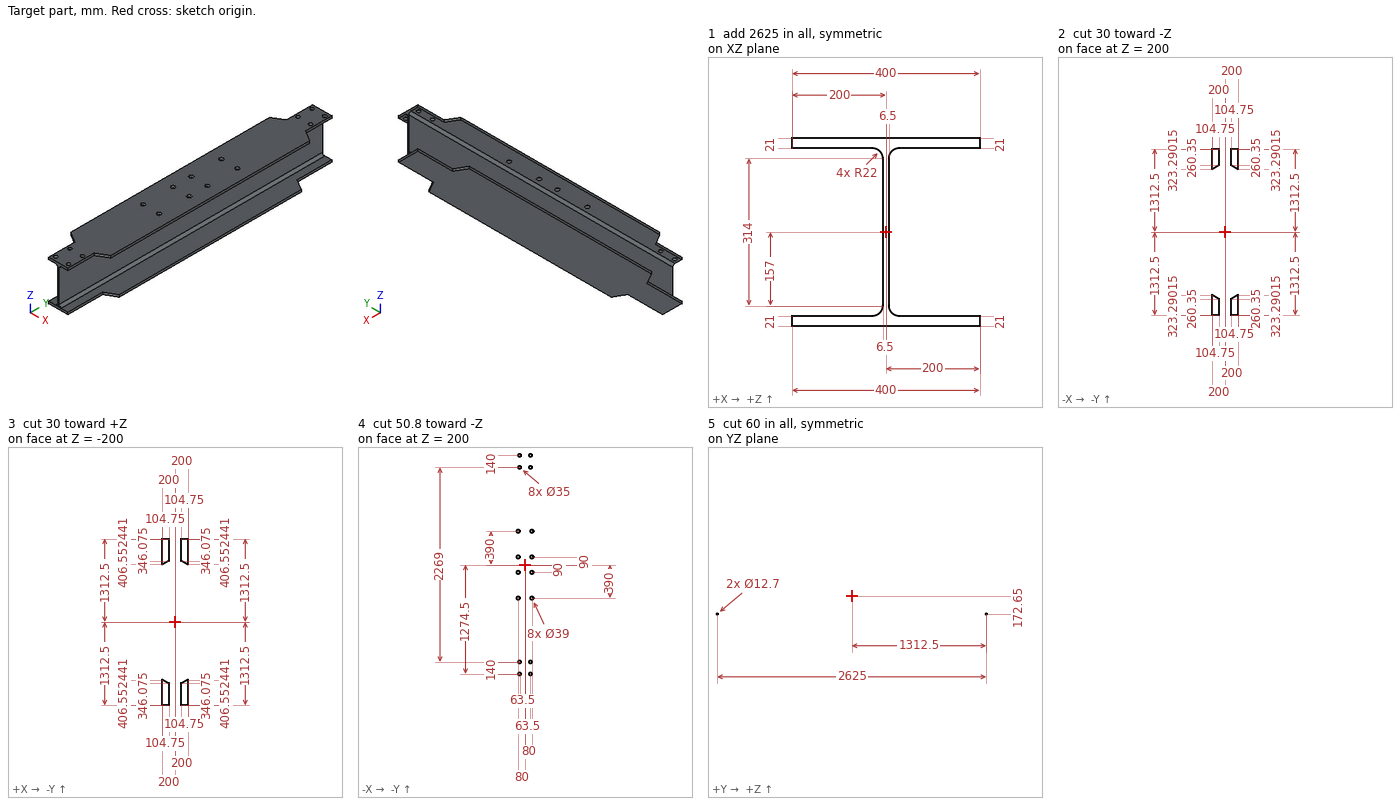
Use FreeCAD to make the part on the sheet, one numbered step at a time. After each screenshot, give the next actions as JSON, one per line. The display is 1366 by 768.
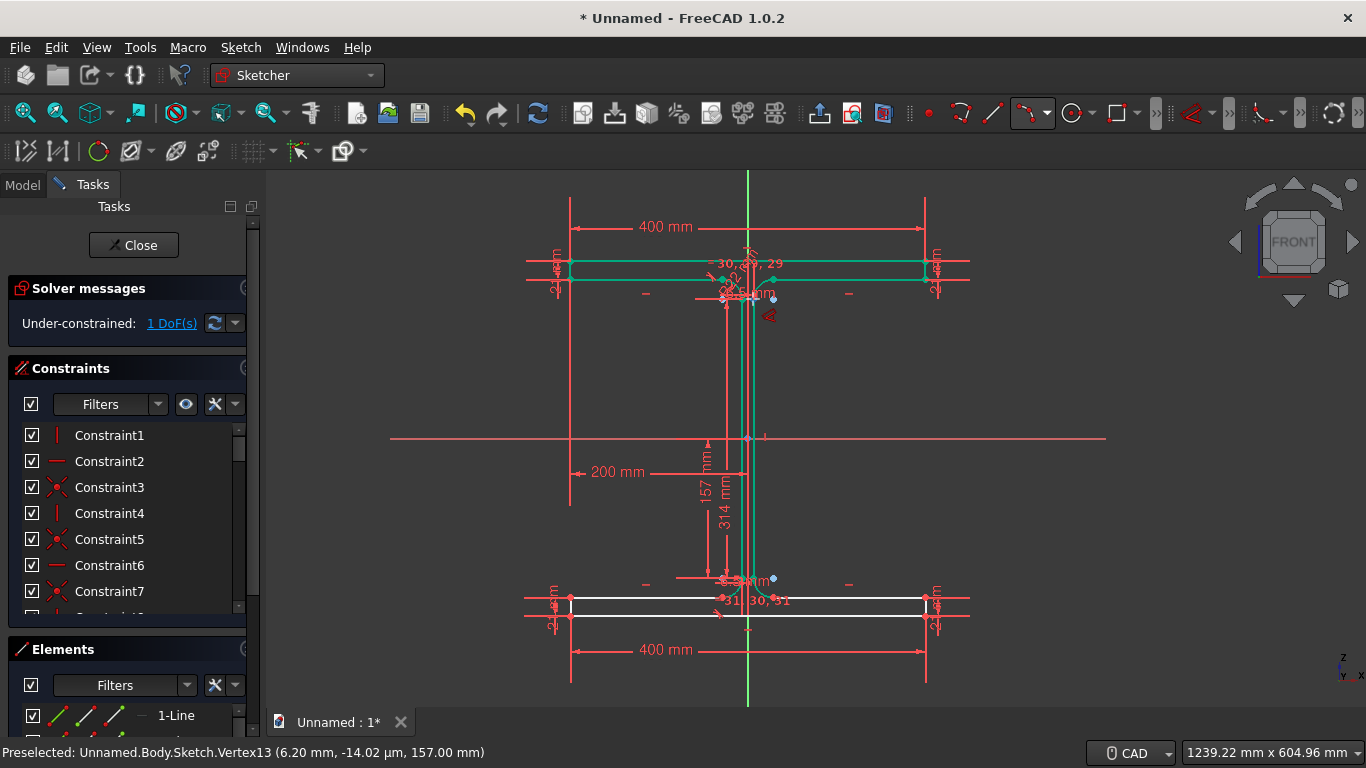
{"action": "left_click", "coordinate": [926, 598]}
{"action": "left_click", "coordinate": [837, 632]}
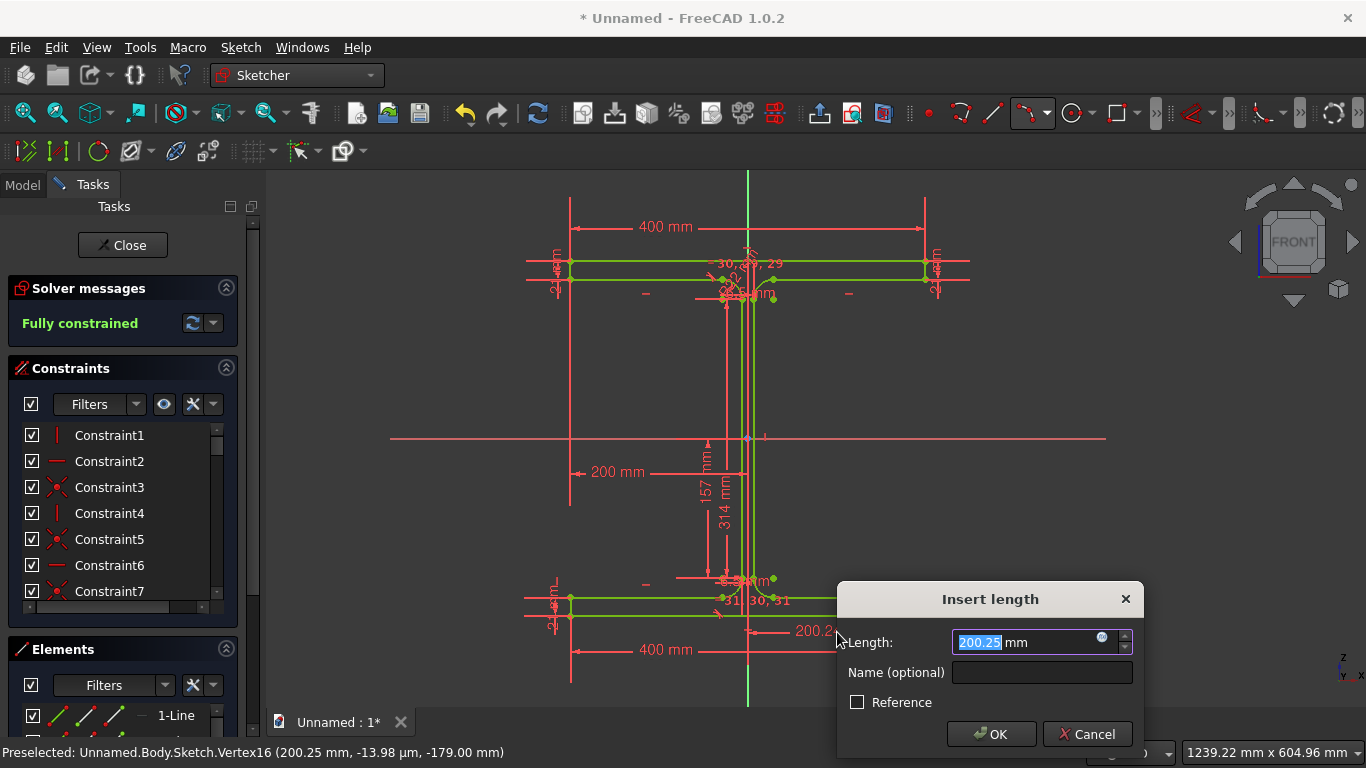
{"action": "type", "text": "200"}
{"action": "key", "text": "Return"}
{"action": "key", "text": "Escape"}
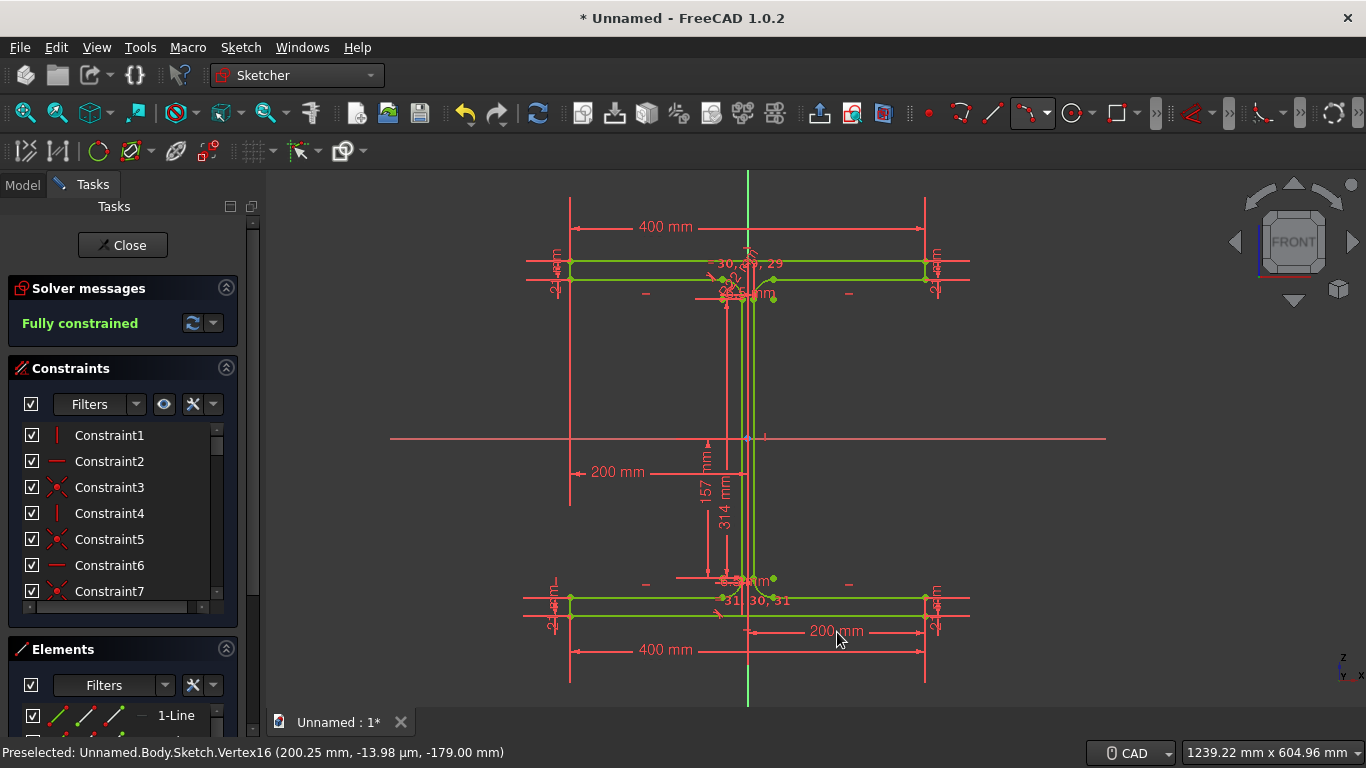
{"action": "left_click", "coordinate": [123, 245]}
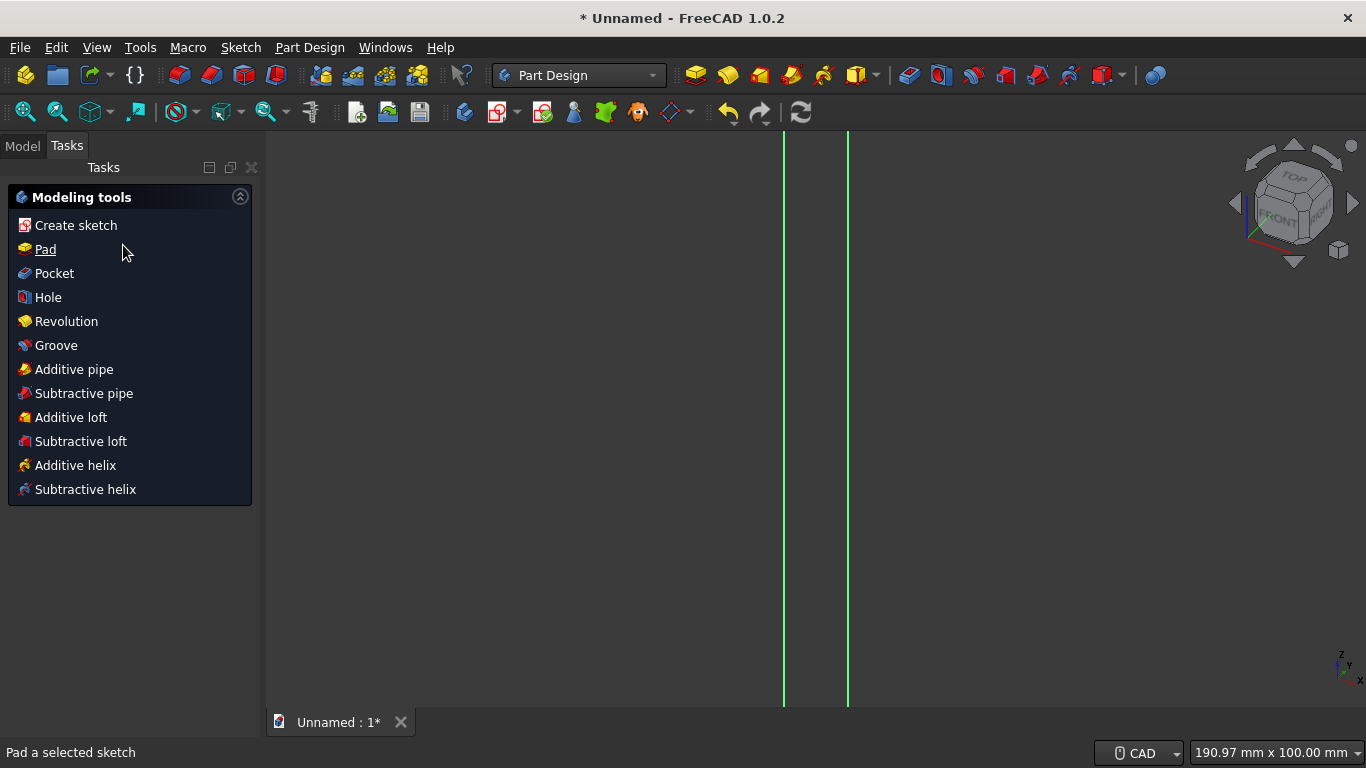
{"action": "left_click", "coordinate": [696, 76]}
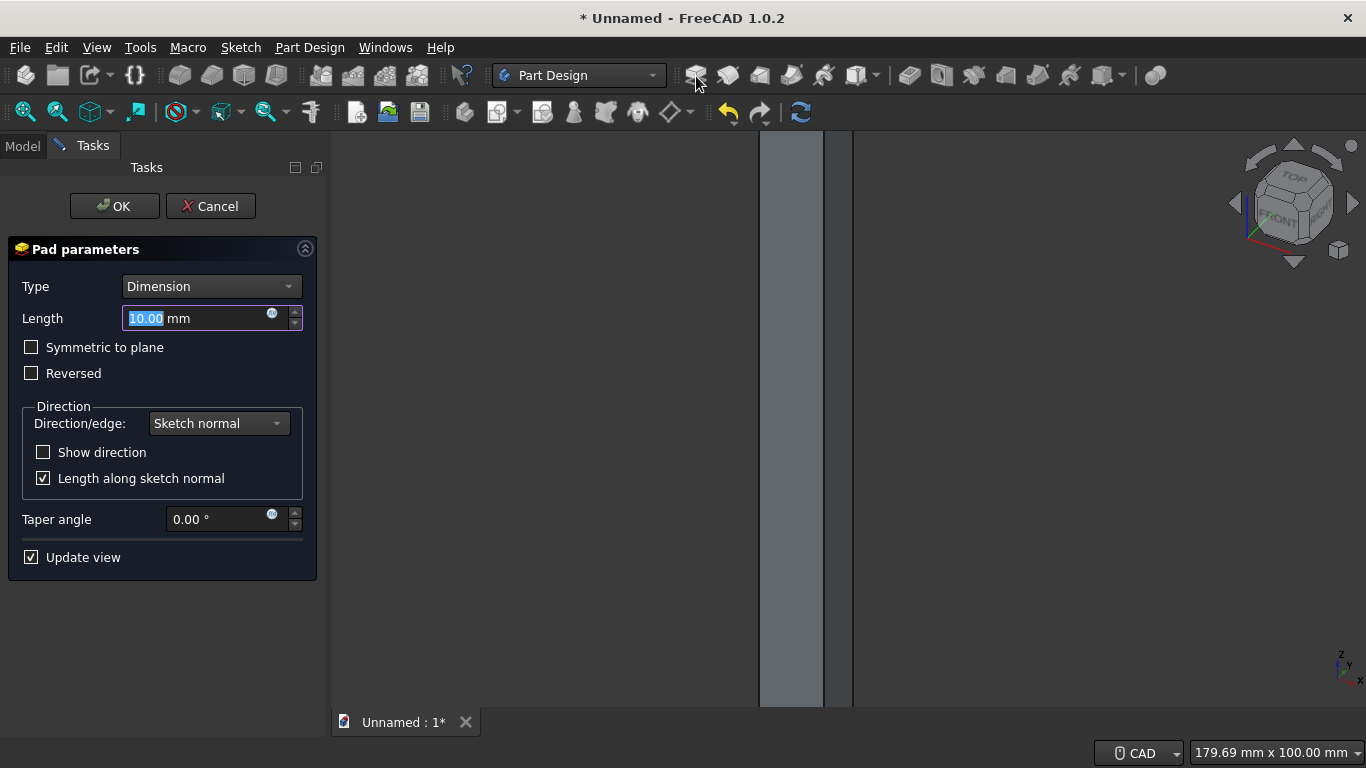
{"action": "type", "text": "2625"}
{"action": "key", "text": "Tab"}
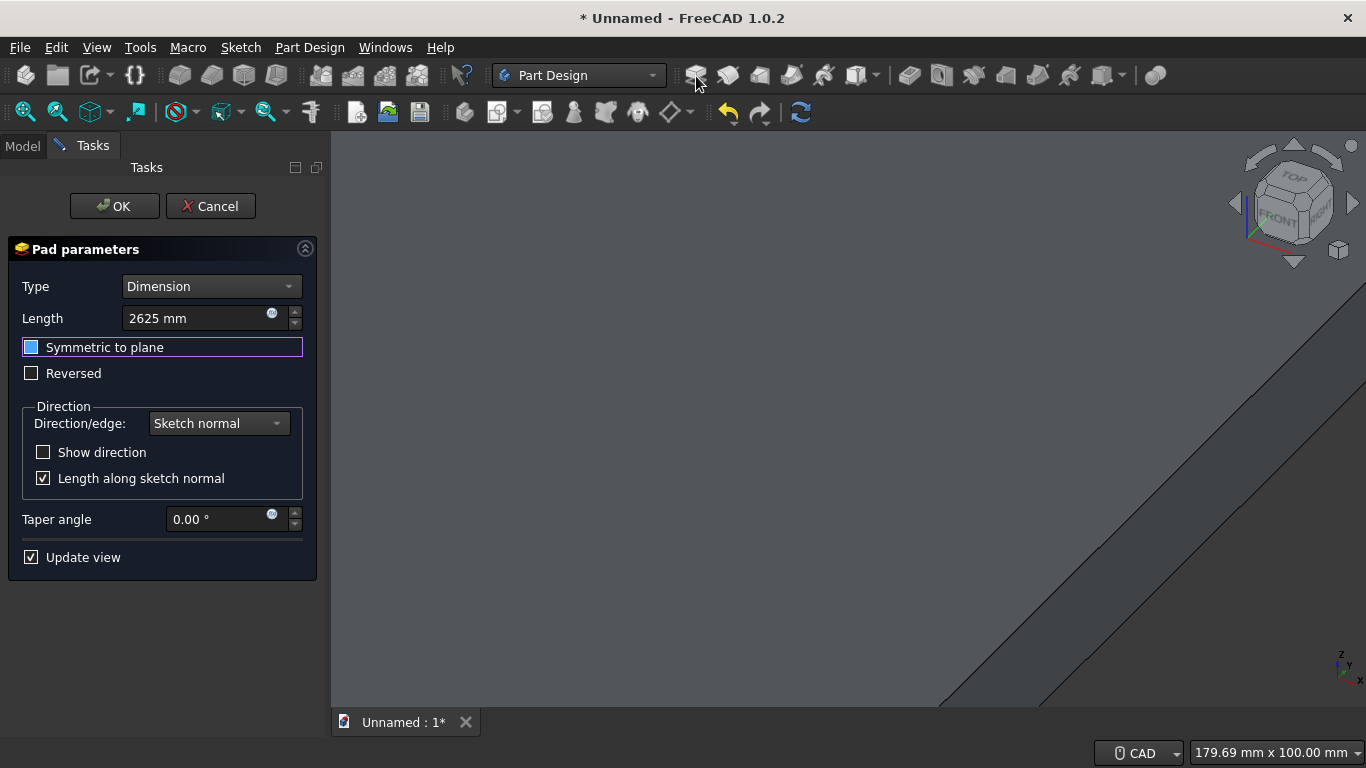
{"action": "left_click", "coordinate": [30, 347]}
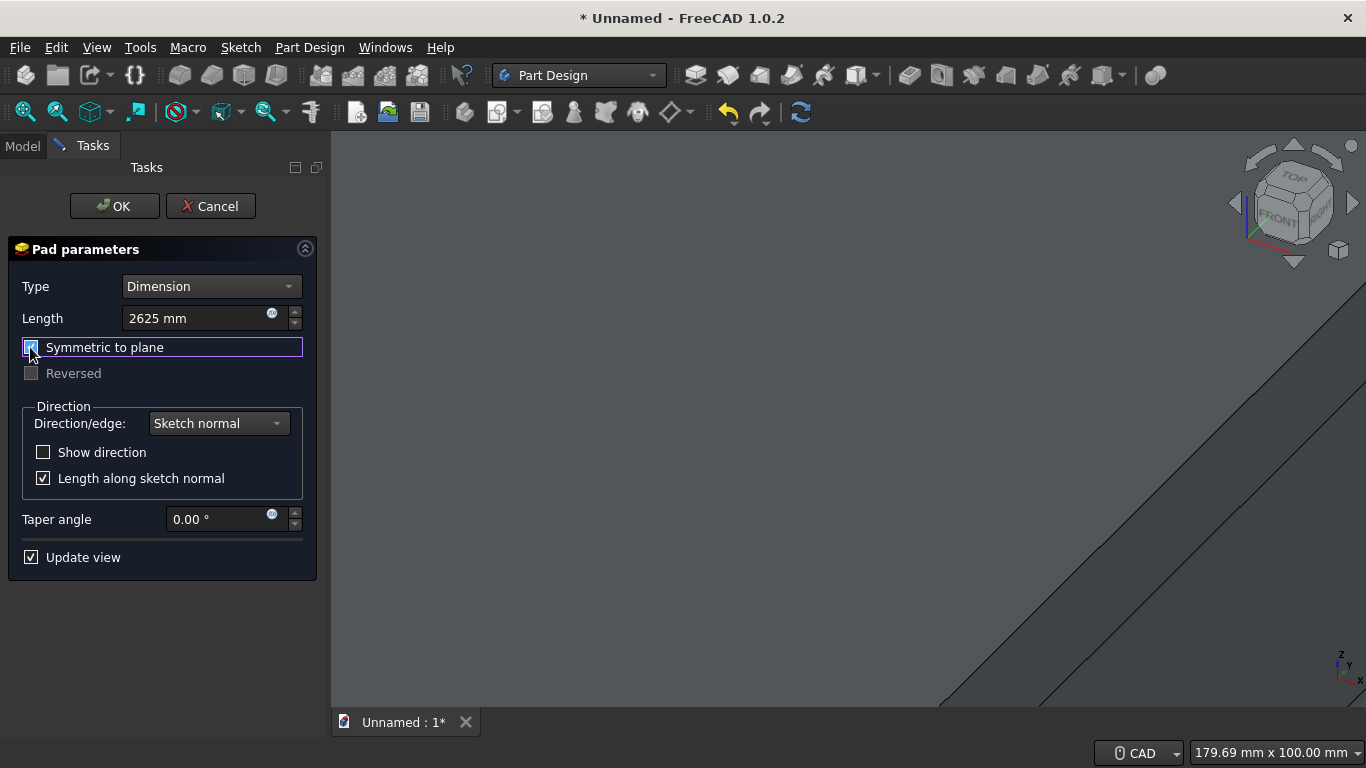
{"action": "left_click", "coordinate": [115, 206]}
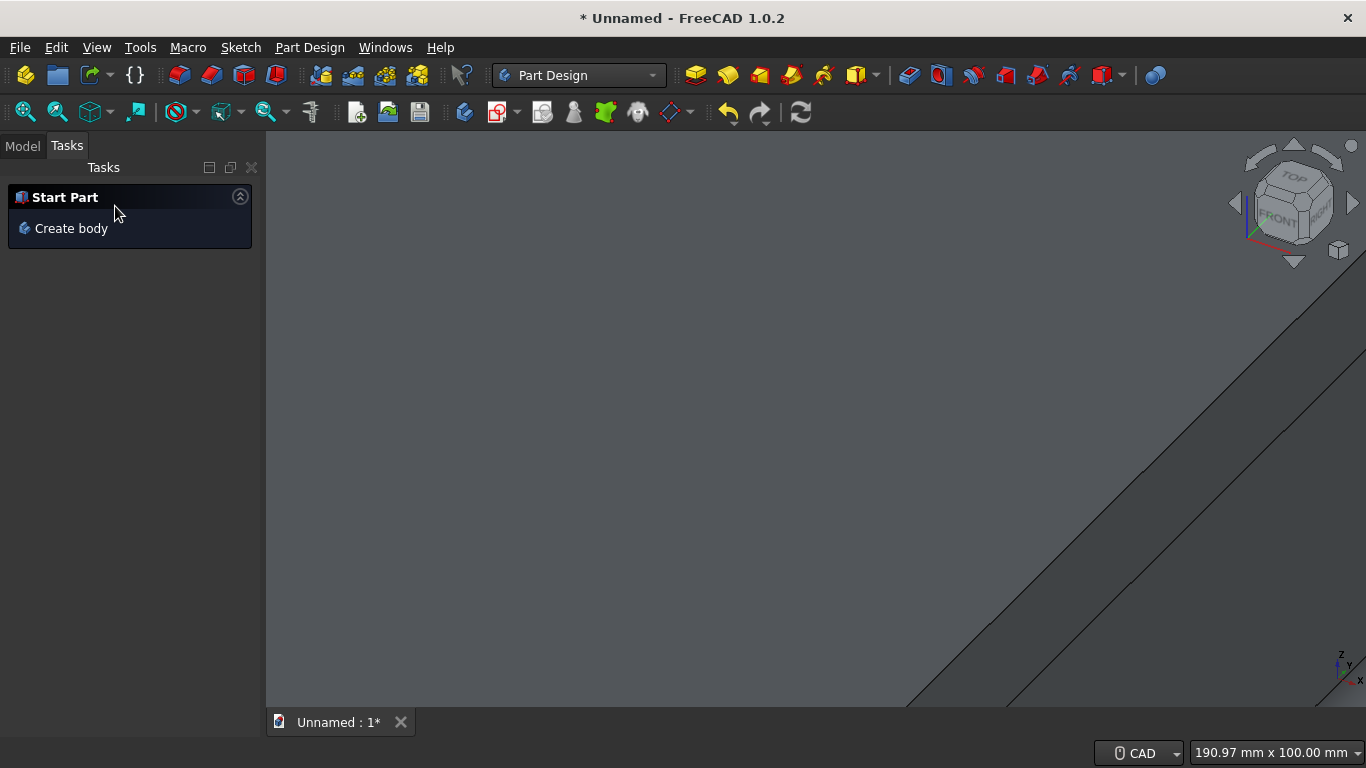
{"action": "left_click", "coordinate": [26, 112]}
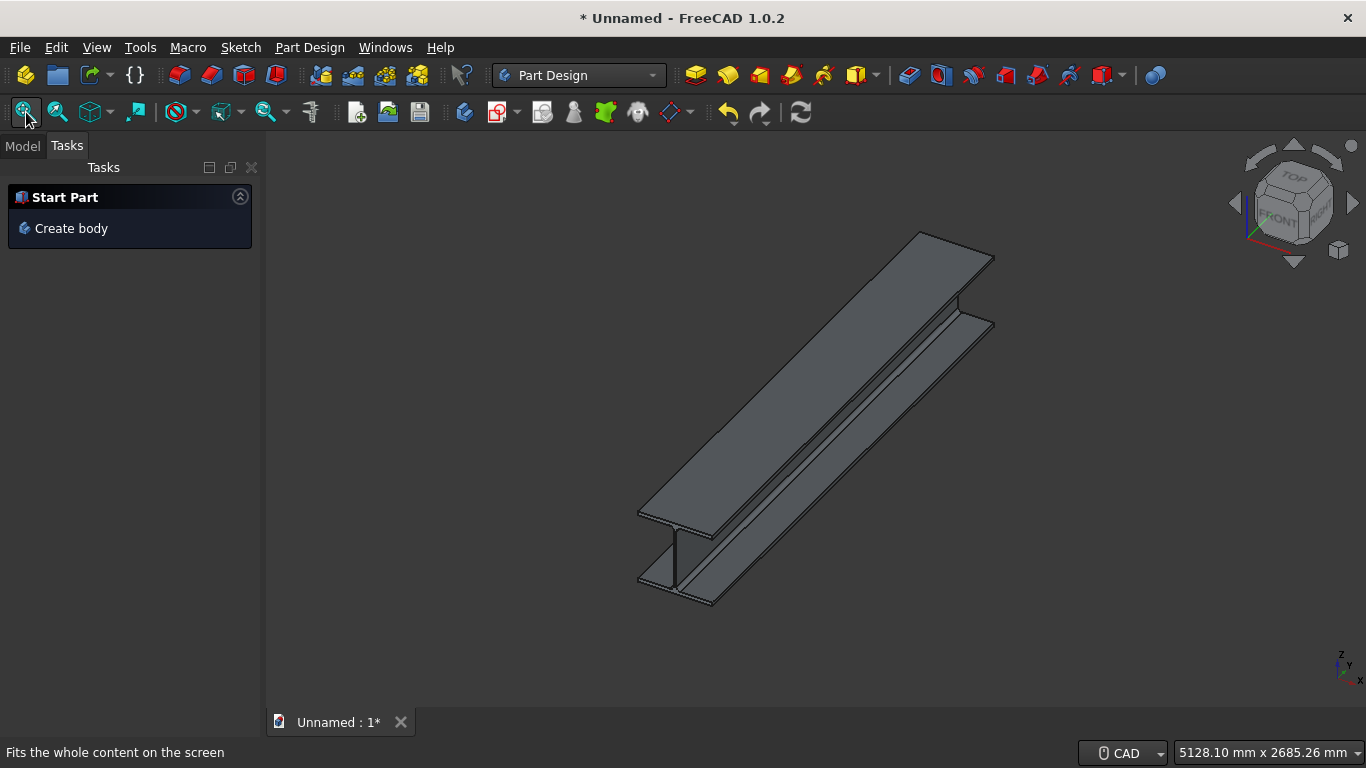
{"action": "left_click", "coordinate": [896, 303]}